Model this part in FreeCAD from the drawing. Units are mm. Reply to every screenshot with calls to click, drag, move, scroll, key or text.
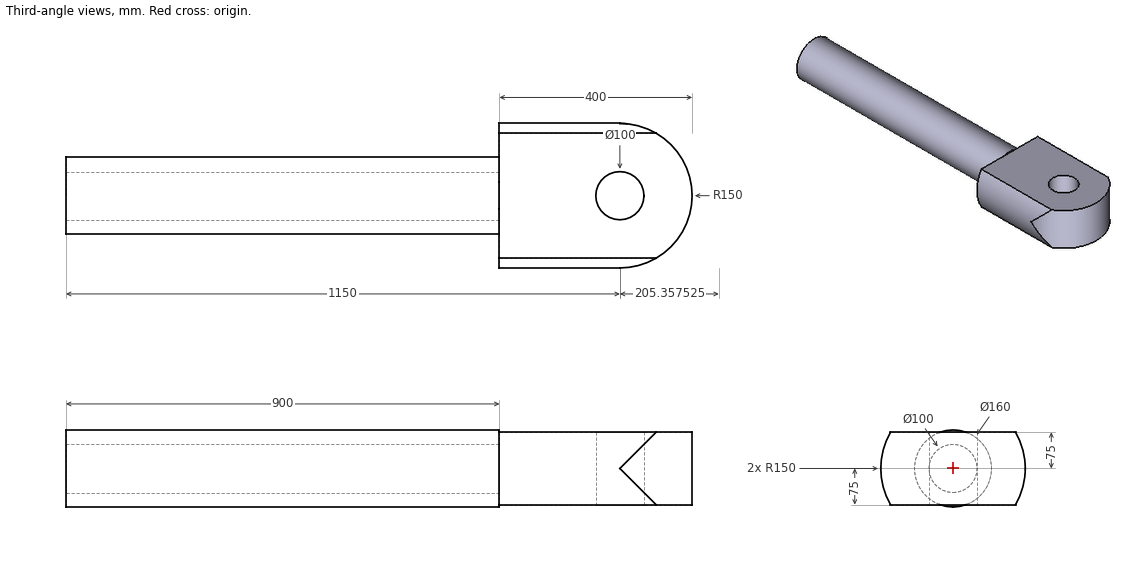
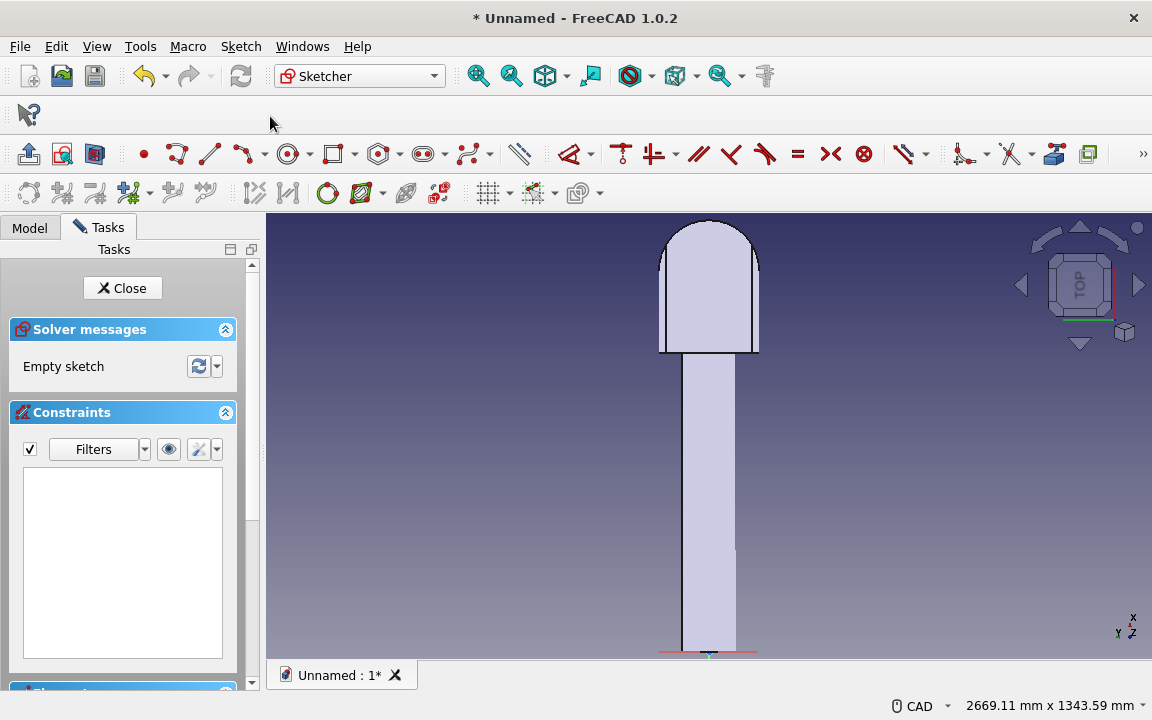
key(q)
key(s)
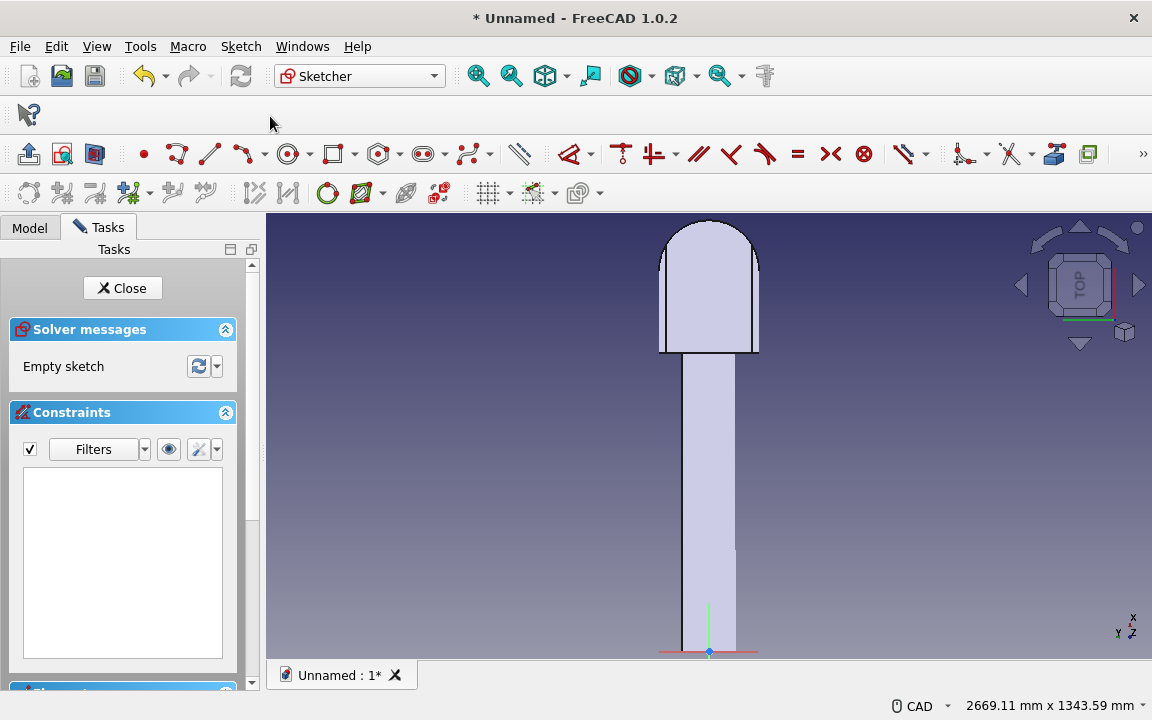
scroll(718, 249, up, 11)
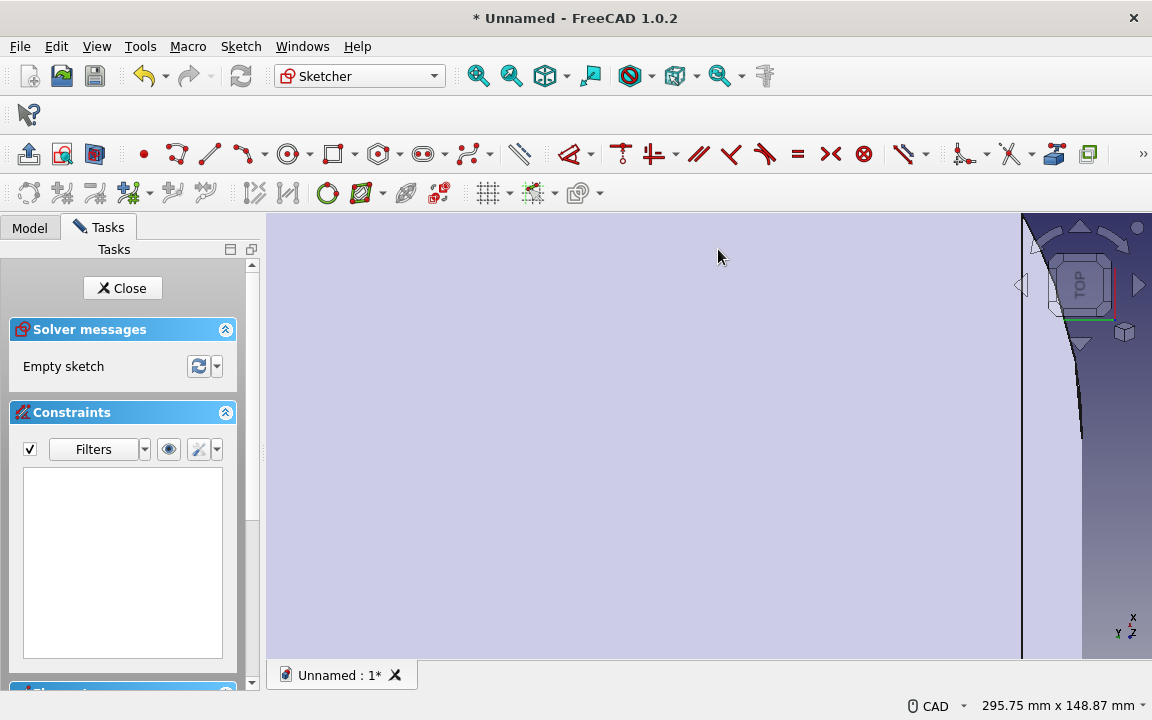
key(g)
key(c)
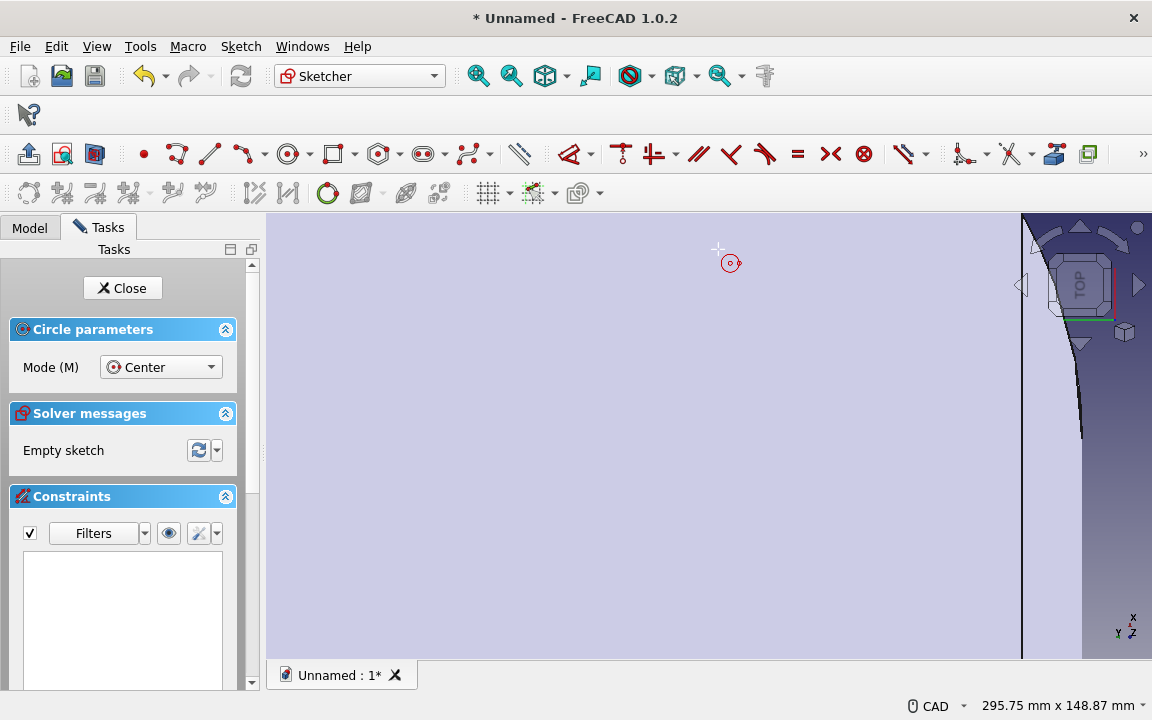
click(633, 438)
move(739, 332)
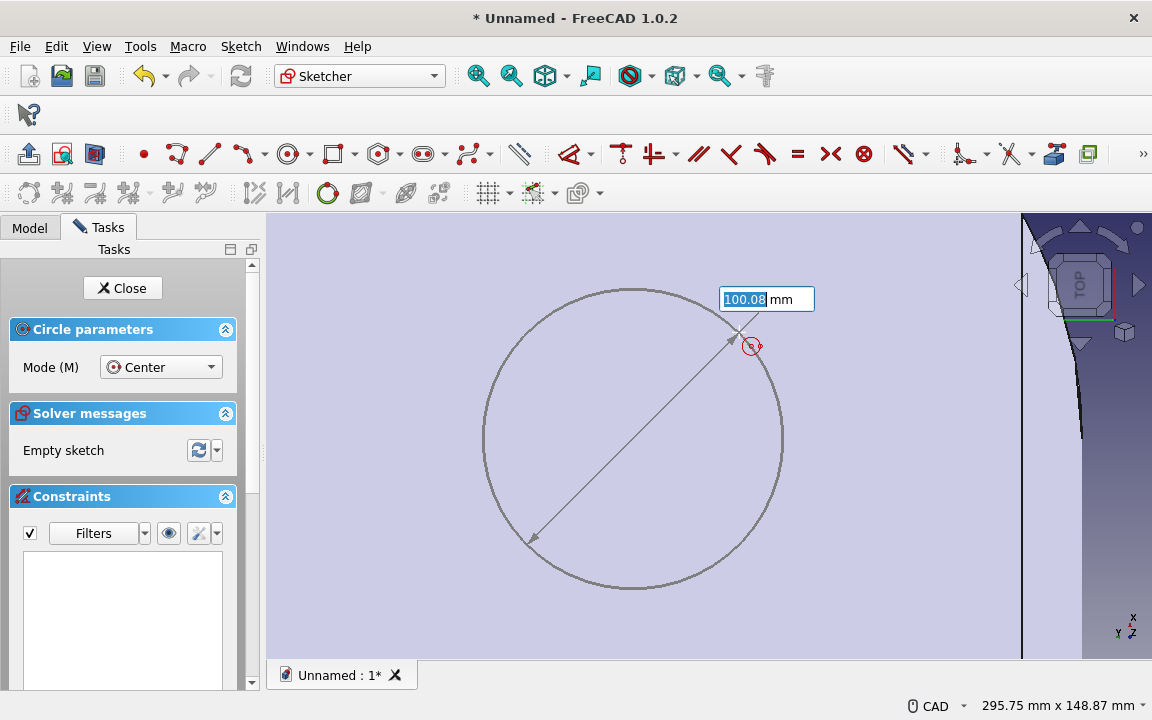
text(100)
key(Return)
key(Escape)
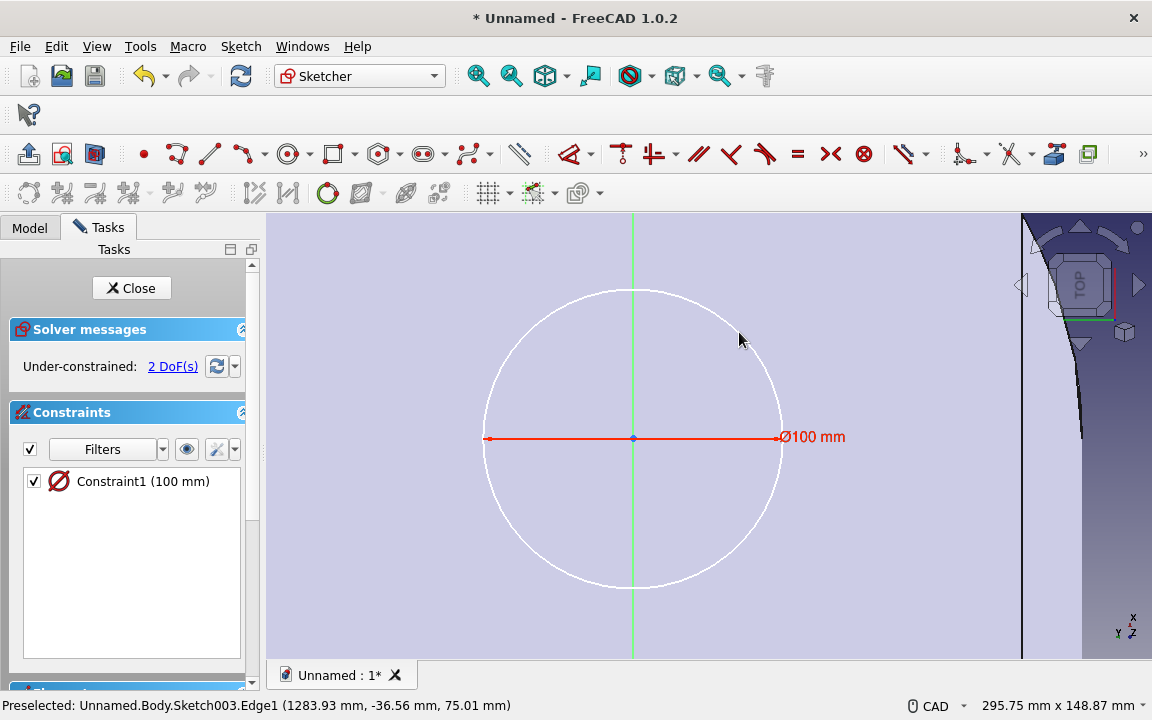
click(633, 439)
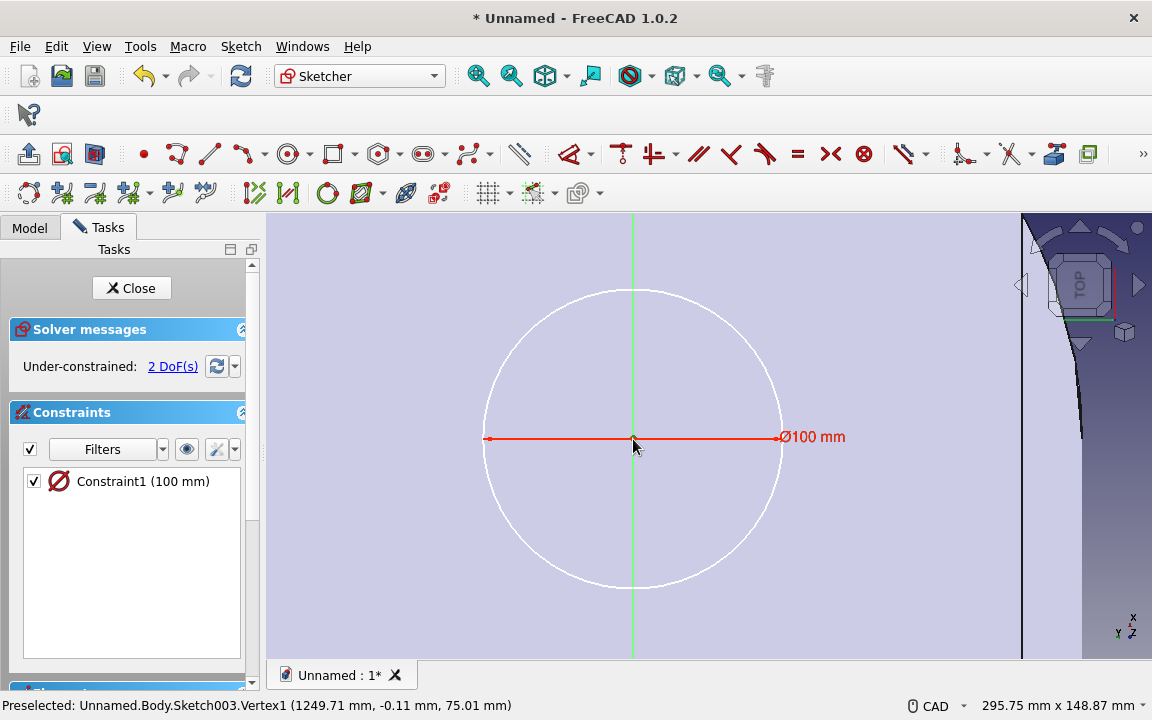
click(633, 547)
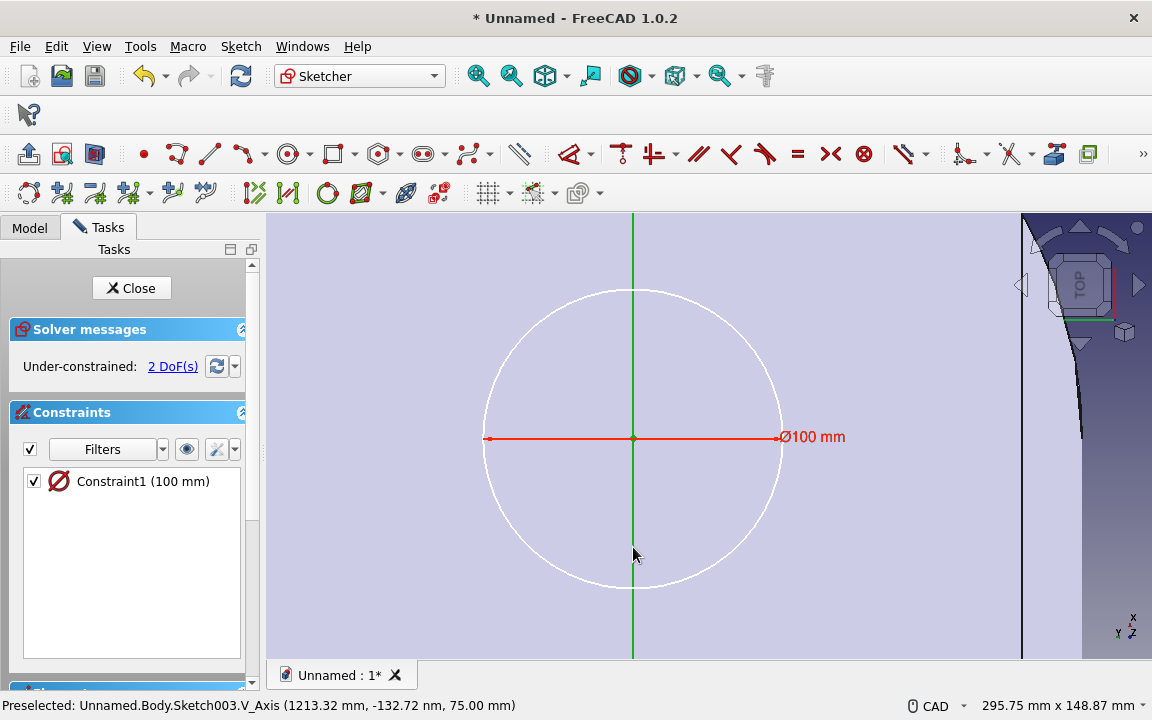
key(c)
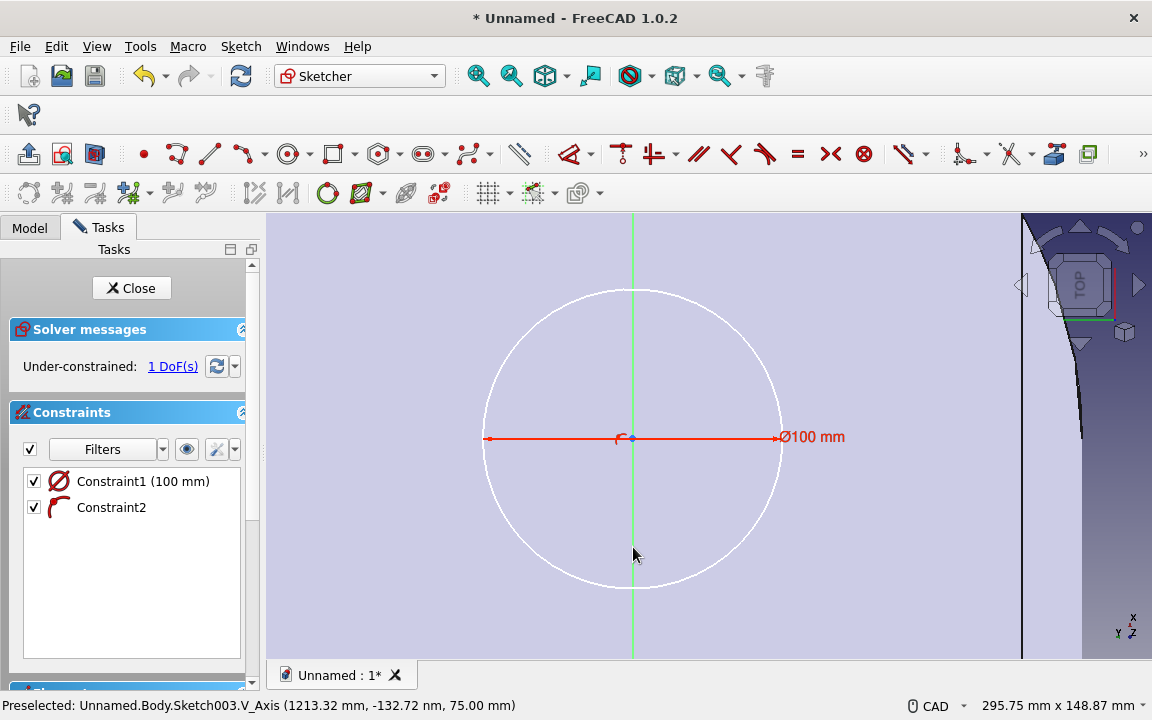
click(568, 154)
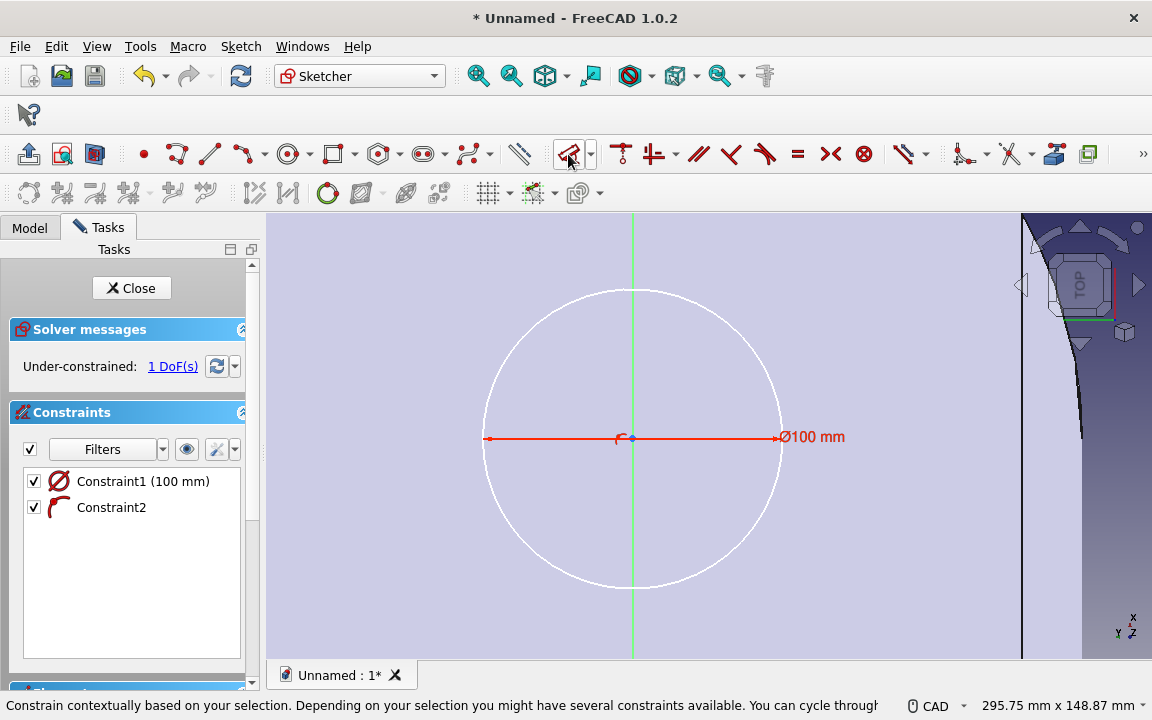
click(633, 439)
click(667, 535)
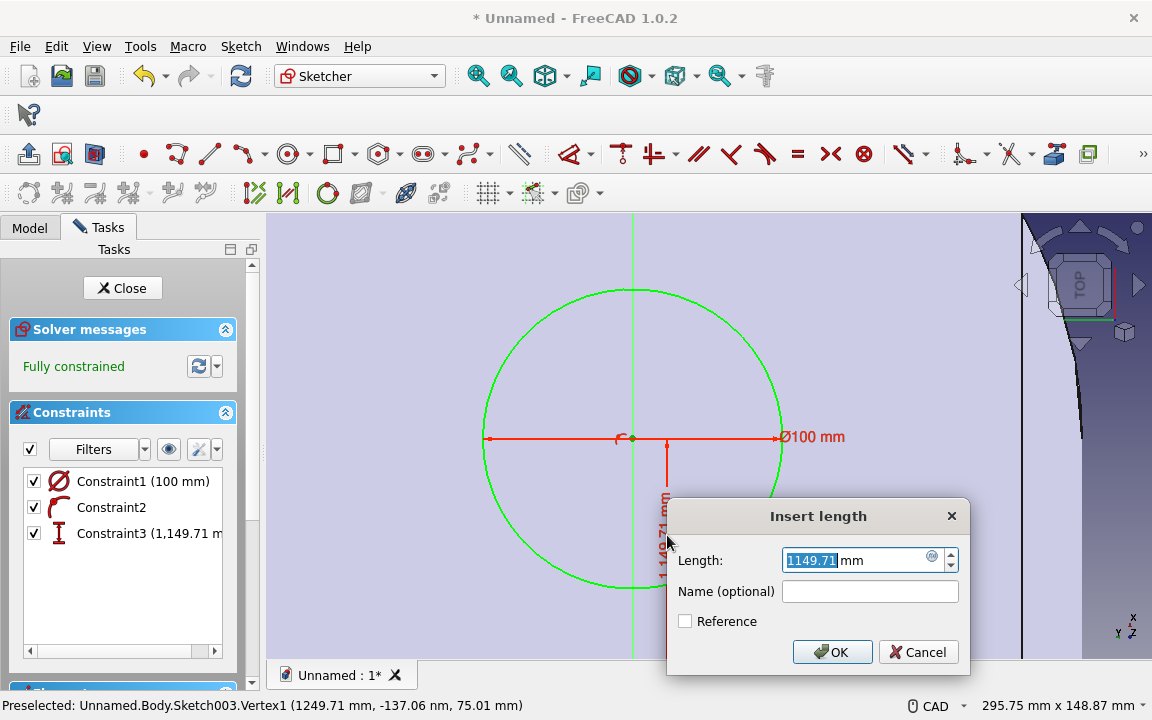
text(1150)
key(Return)
key(Escape)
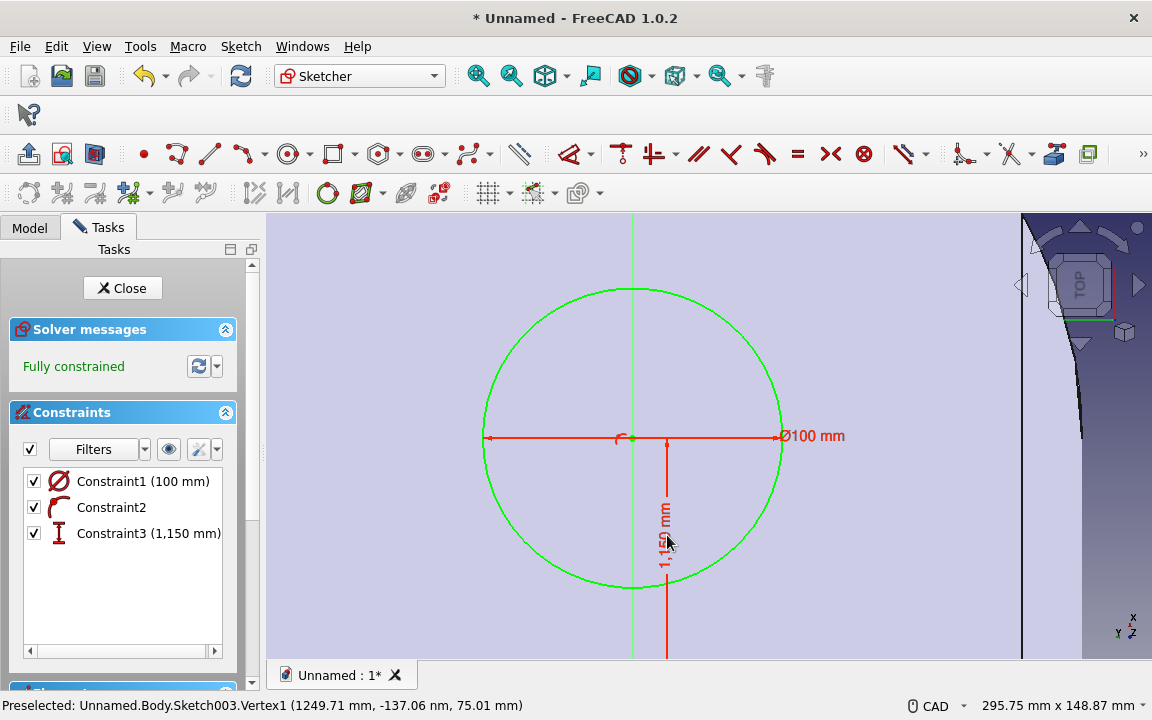
click(123, 288)